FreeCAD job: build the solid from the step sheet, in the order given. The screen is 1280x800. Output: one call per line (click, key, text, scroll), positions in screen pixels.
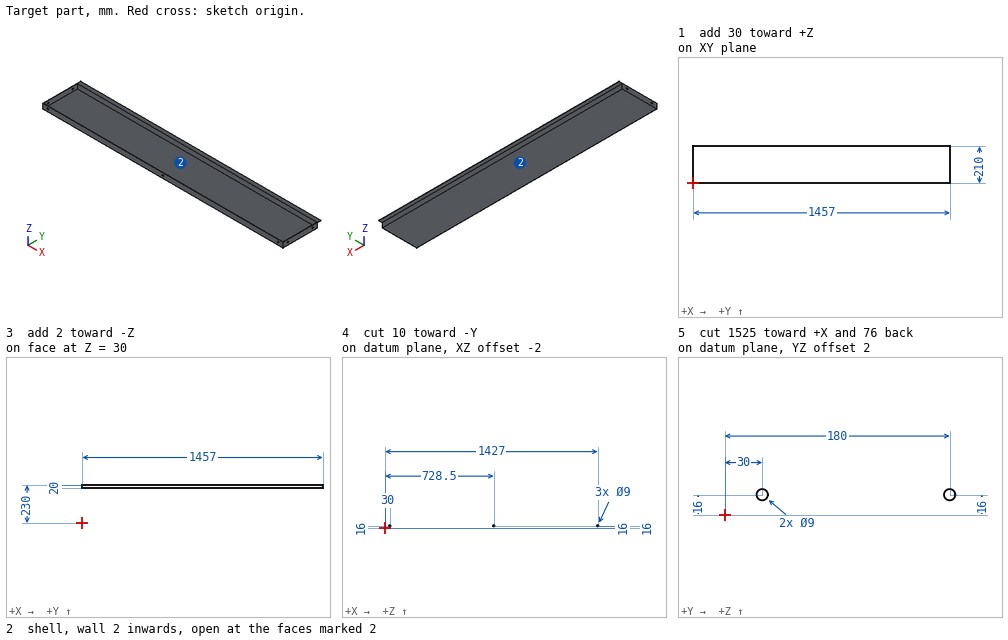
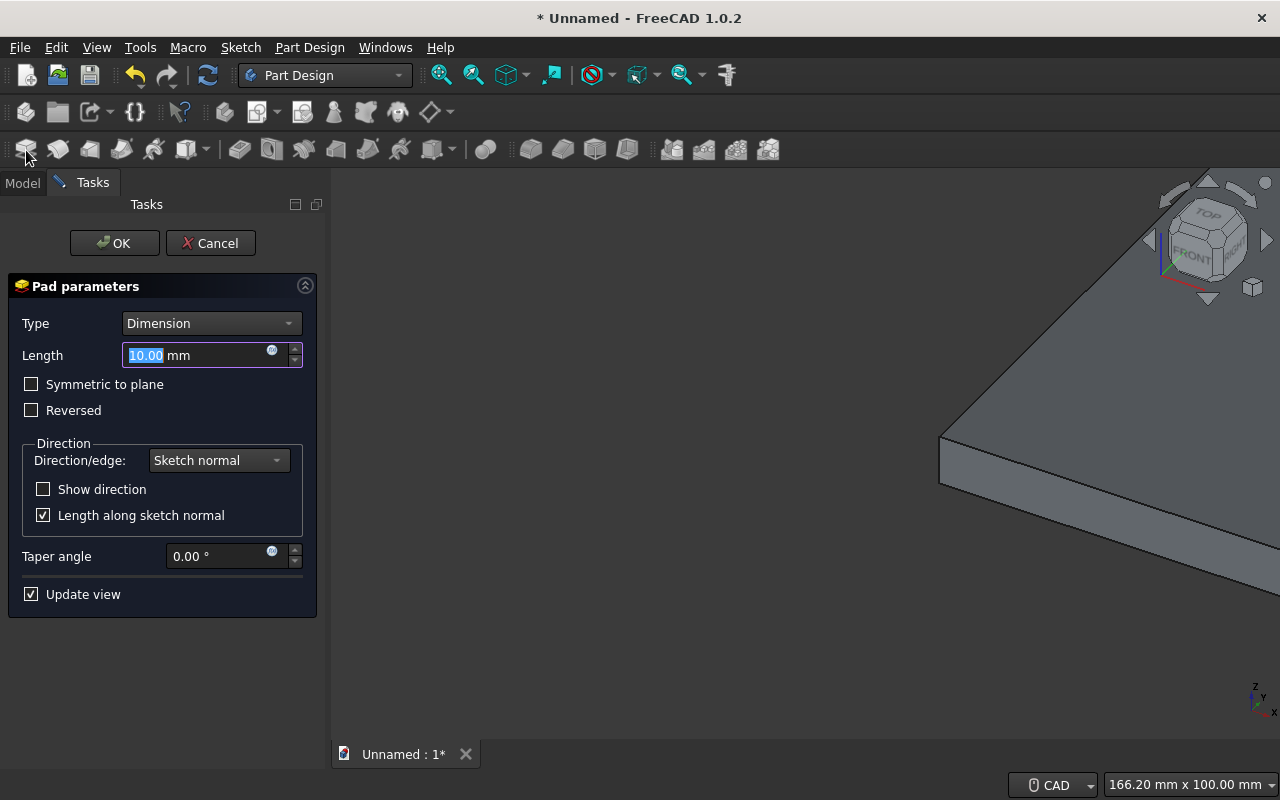
text(30)
key(Tab)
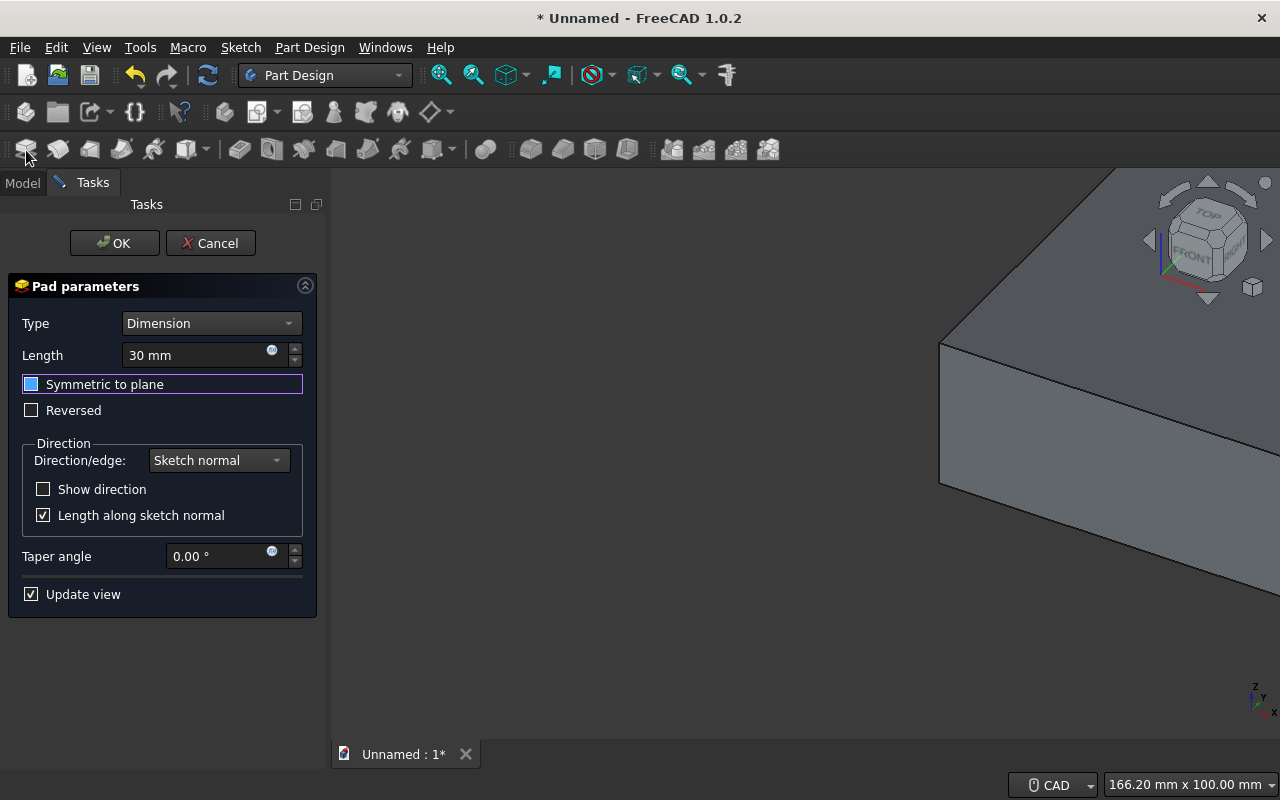
click(115, 243)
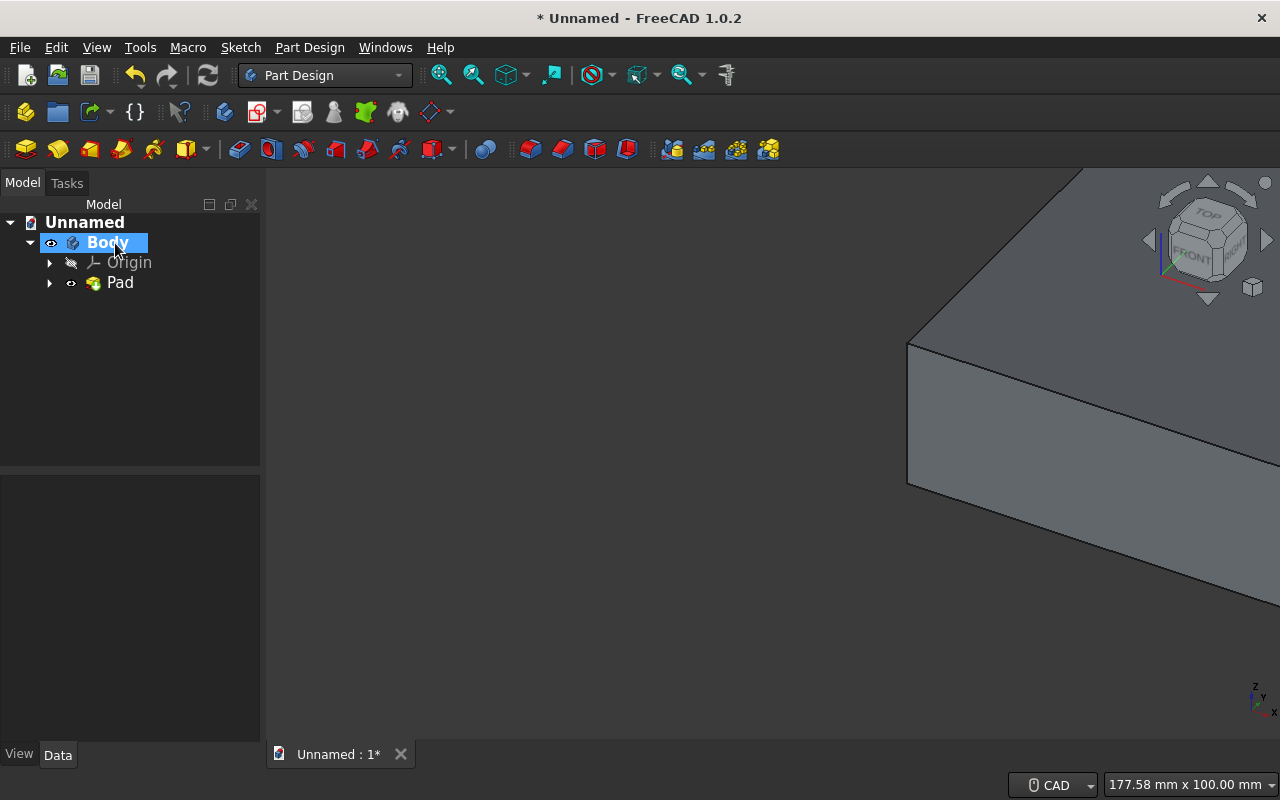
click(442, 76)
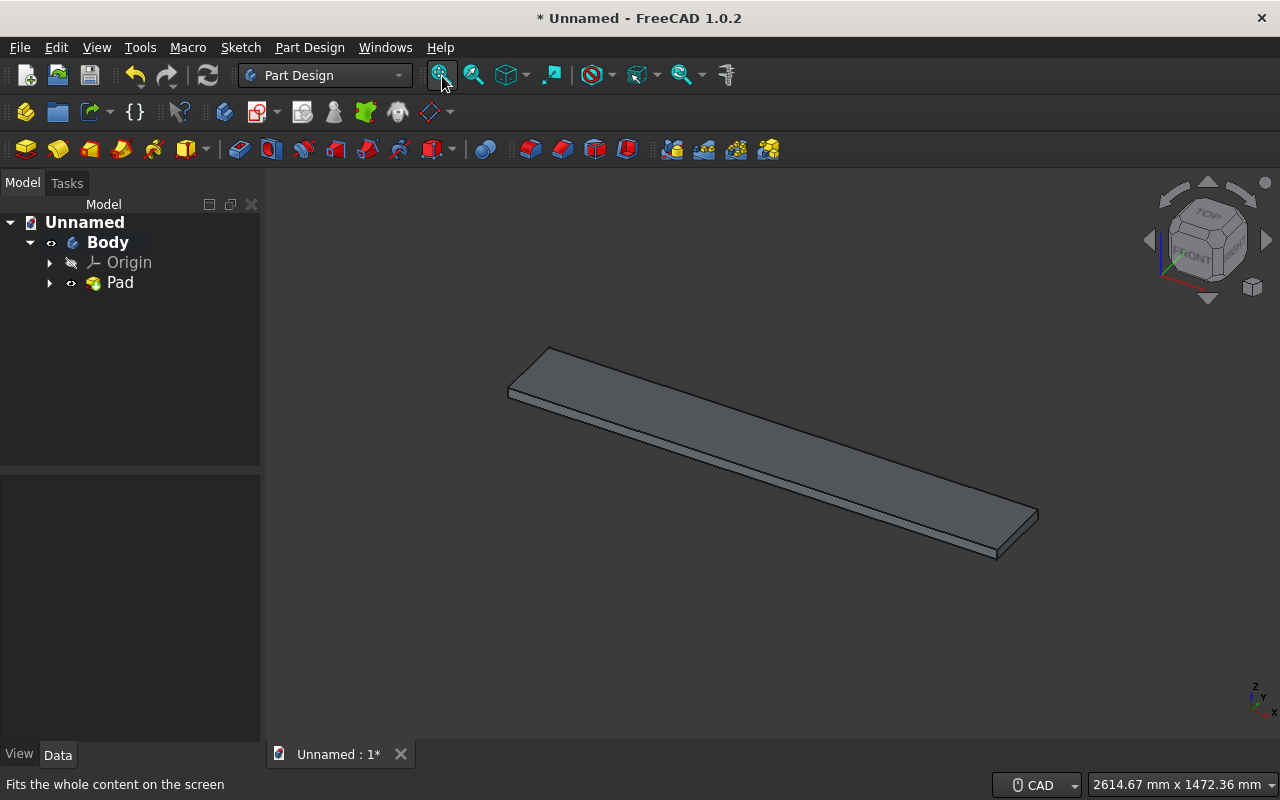
click(913, 494)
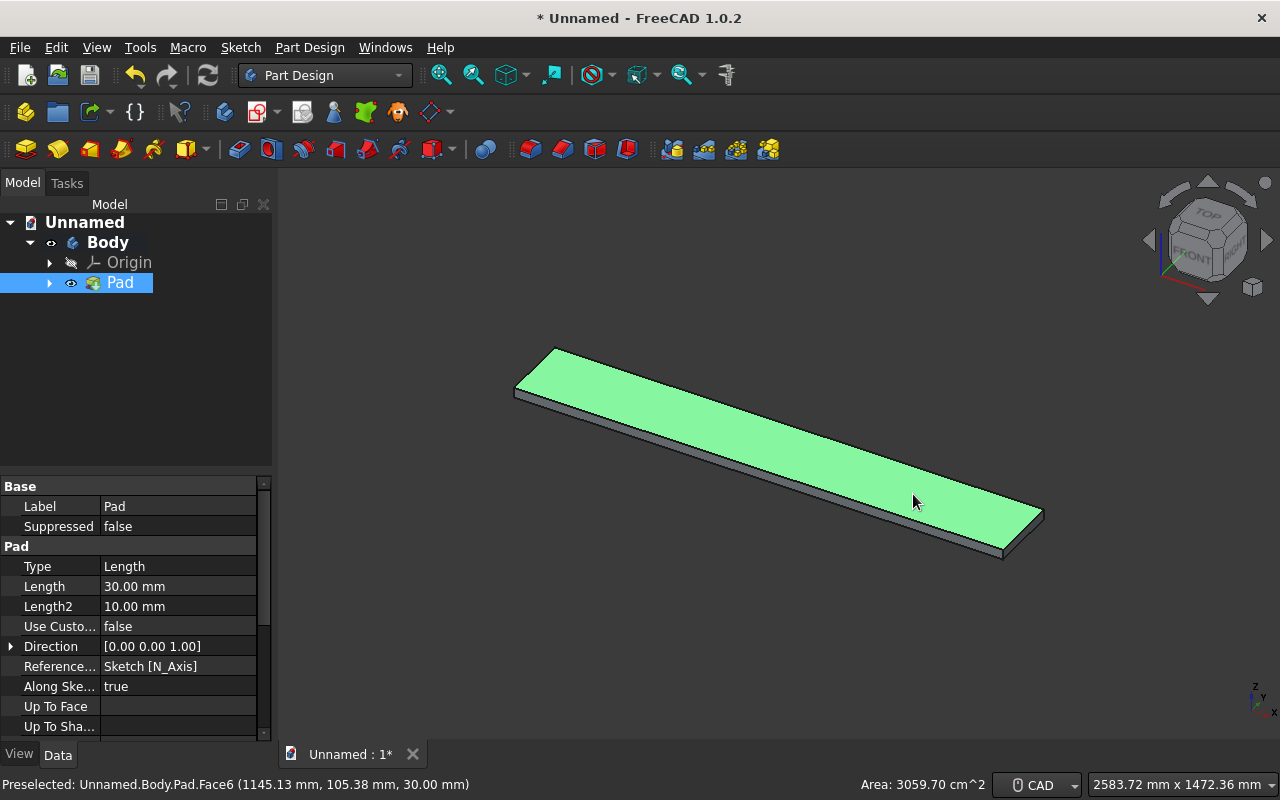
click(628, 150)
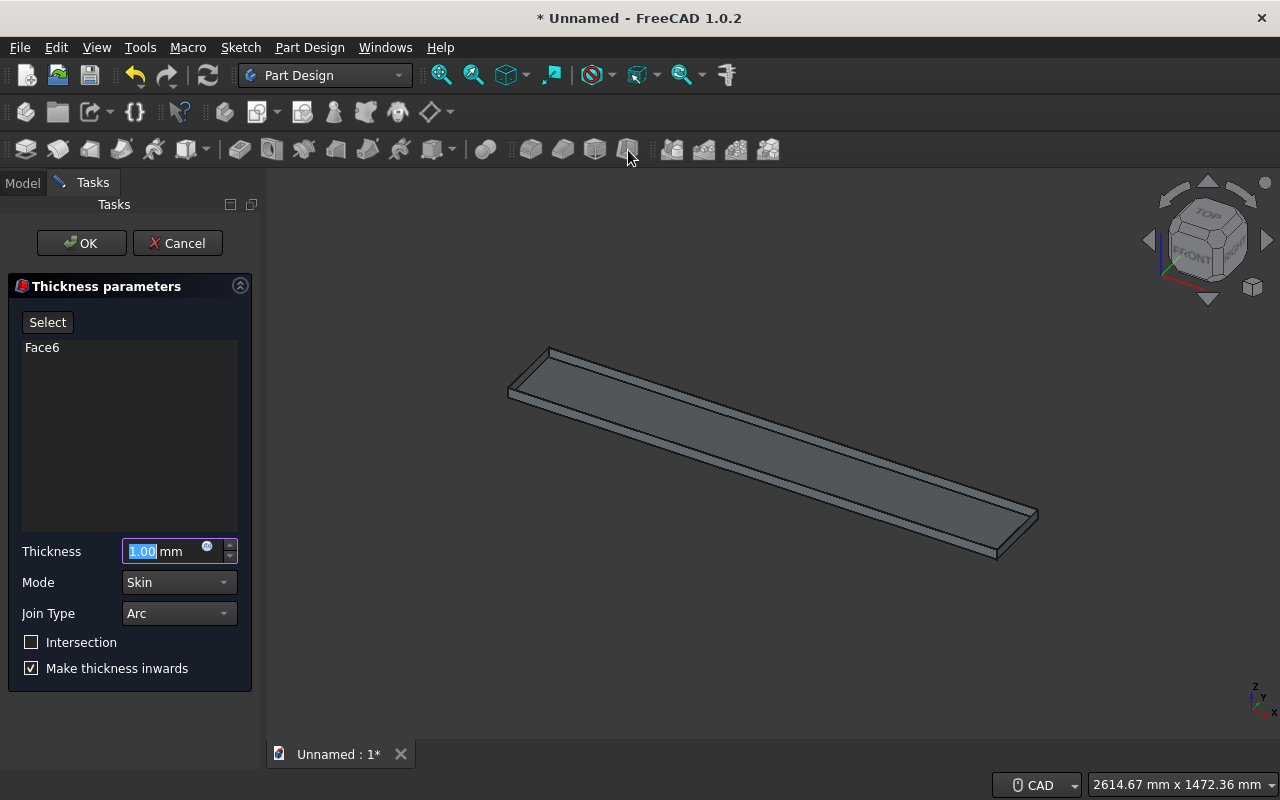
text(2)
key(Tab)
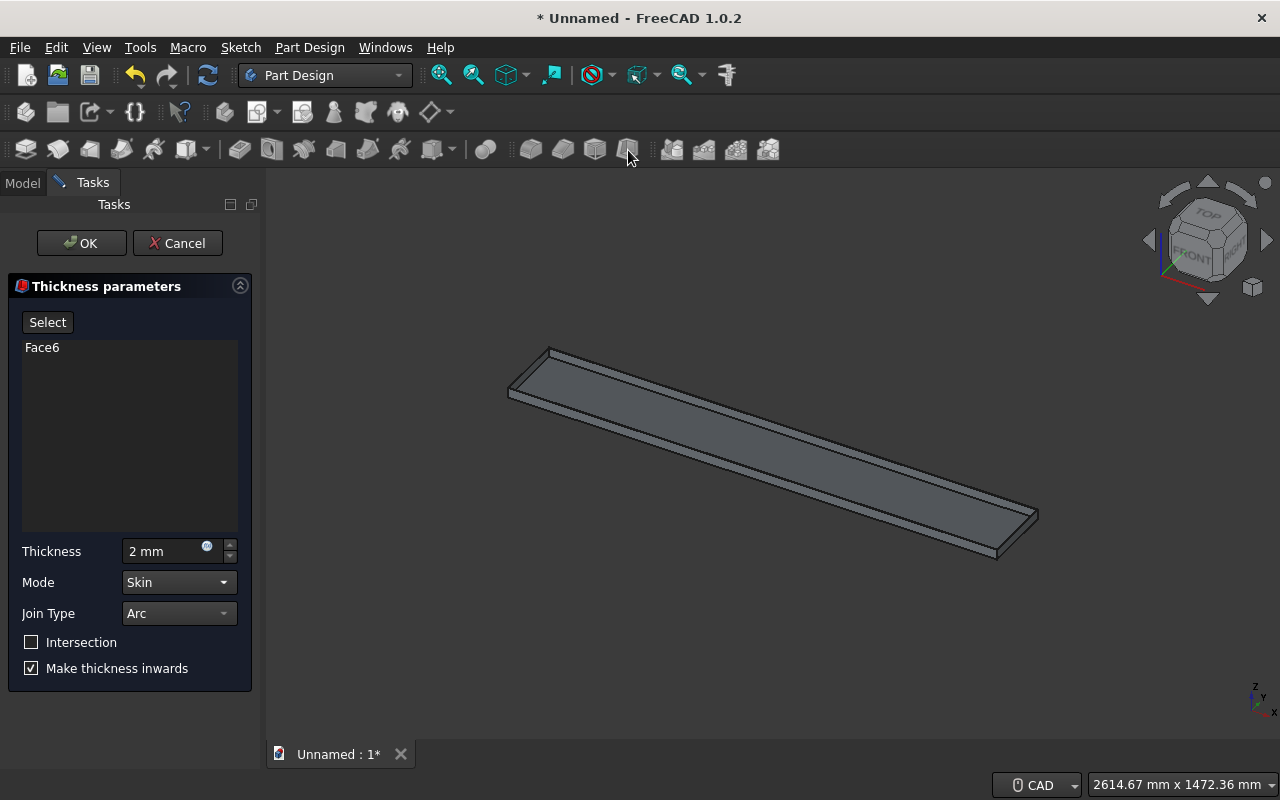
click(180, 614)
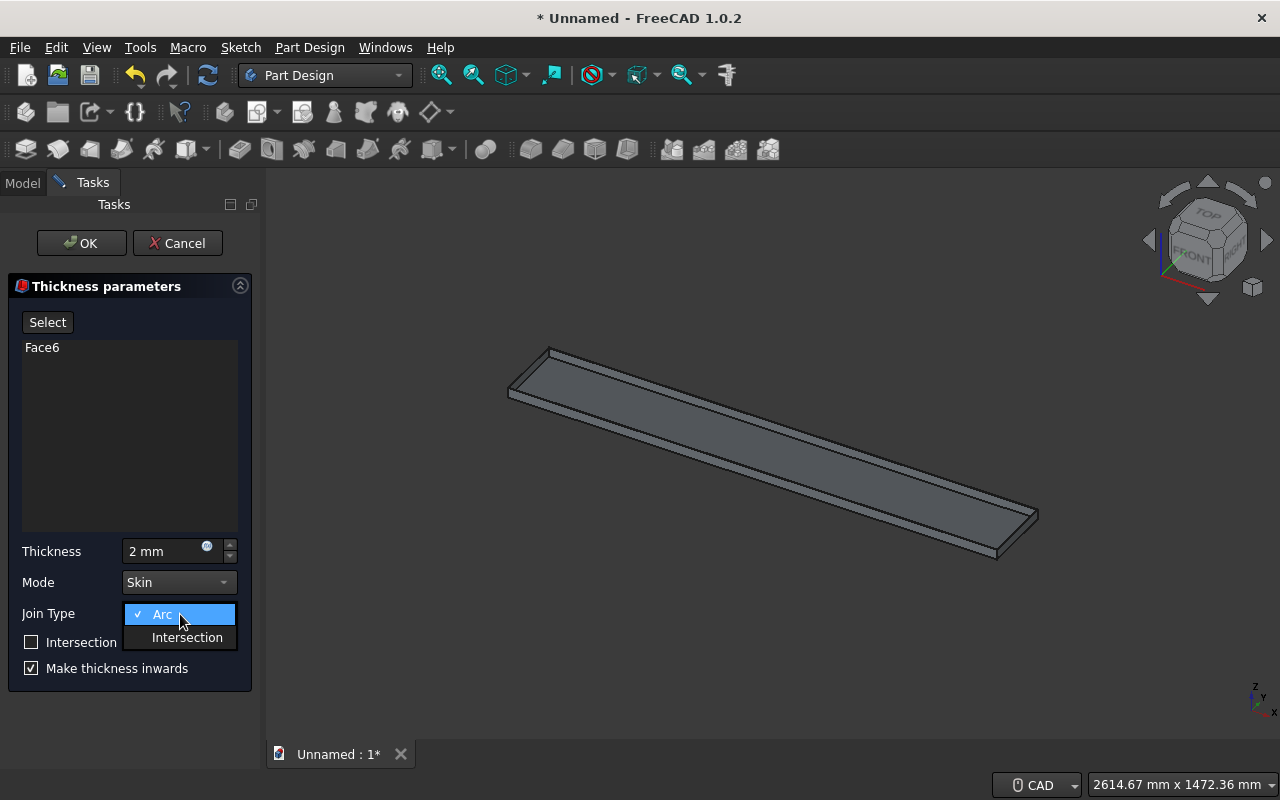
click(179, 638)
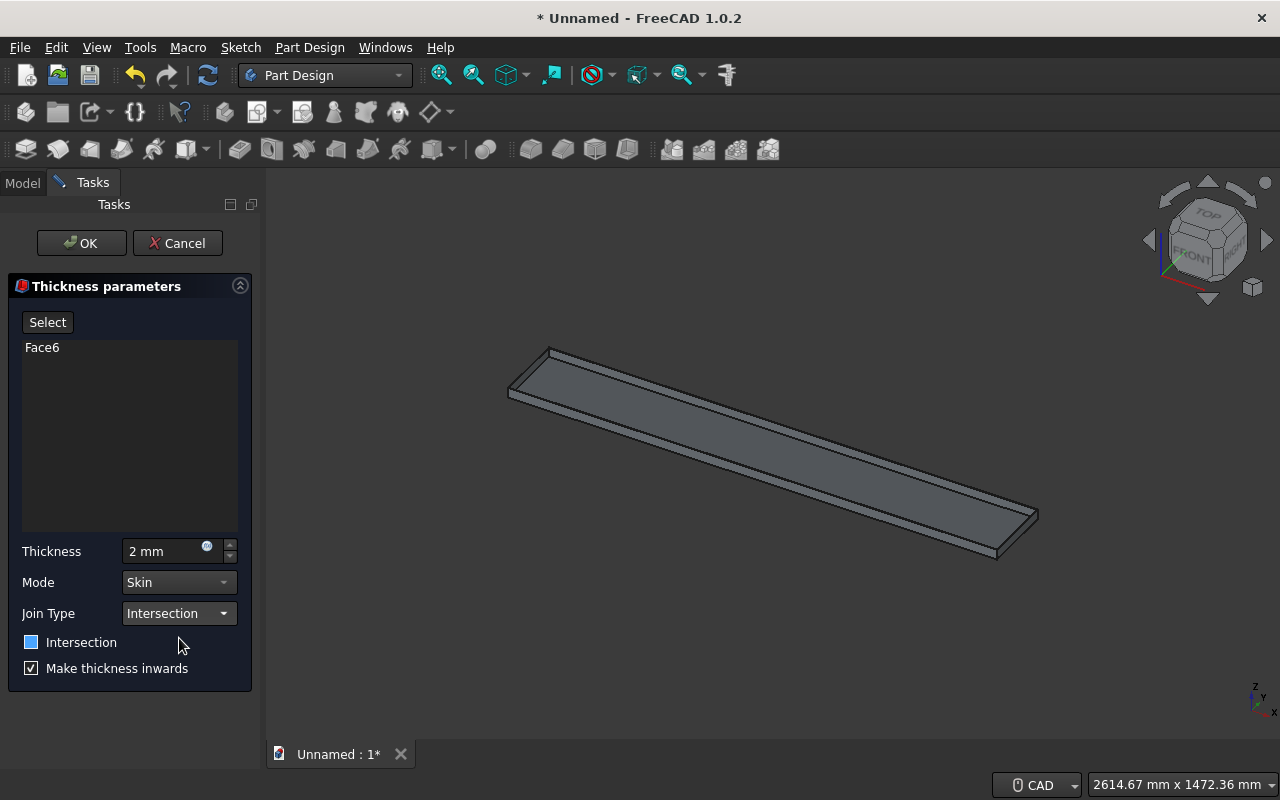
click(82, 243)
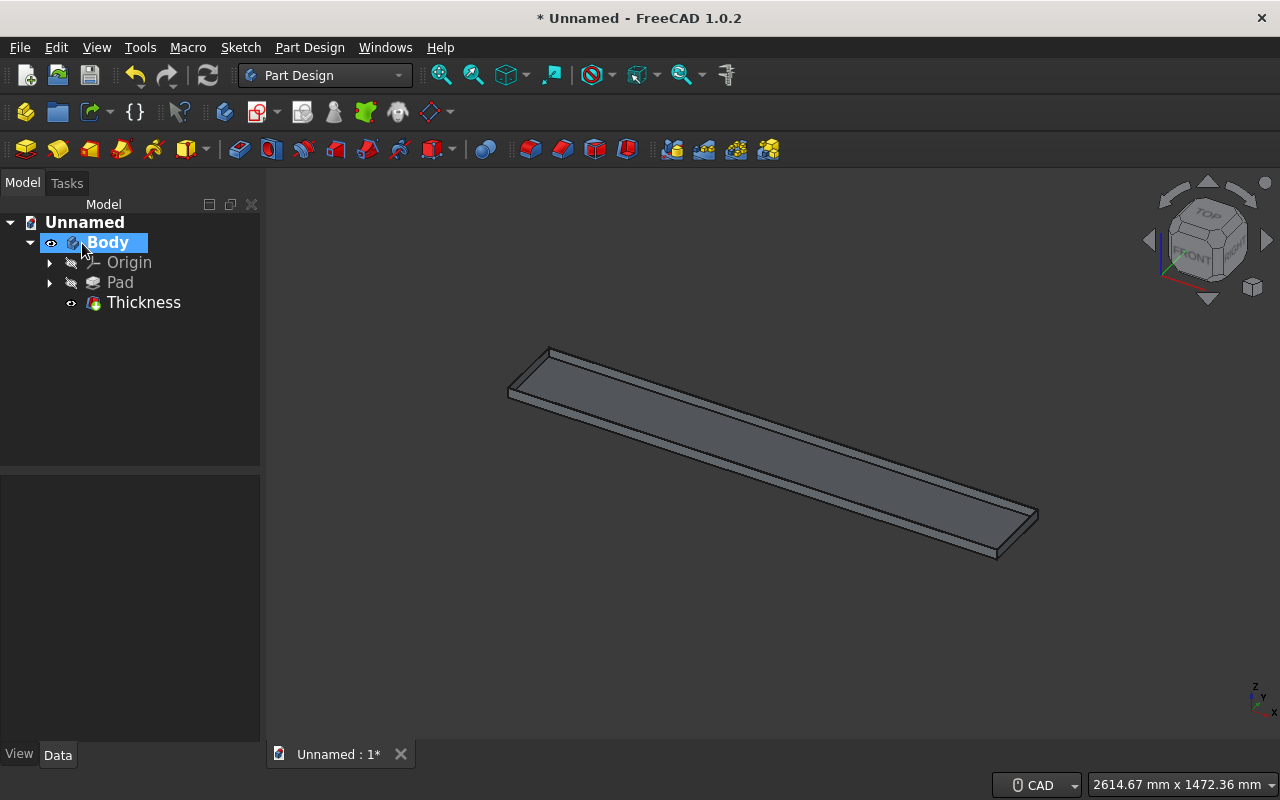
scroll(1024, 522, up, 15)